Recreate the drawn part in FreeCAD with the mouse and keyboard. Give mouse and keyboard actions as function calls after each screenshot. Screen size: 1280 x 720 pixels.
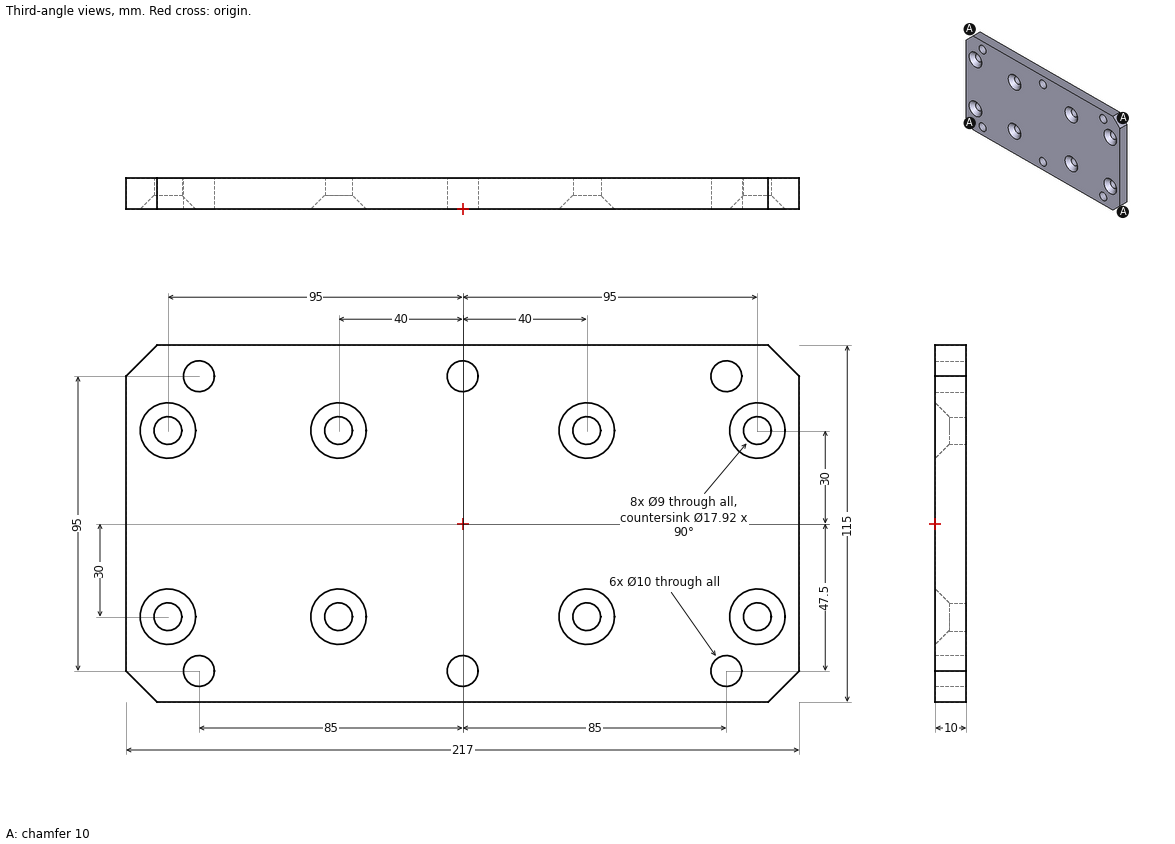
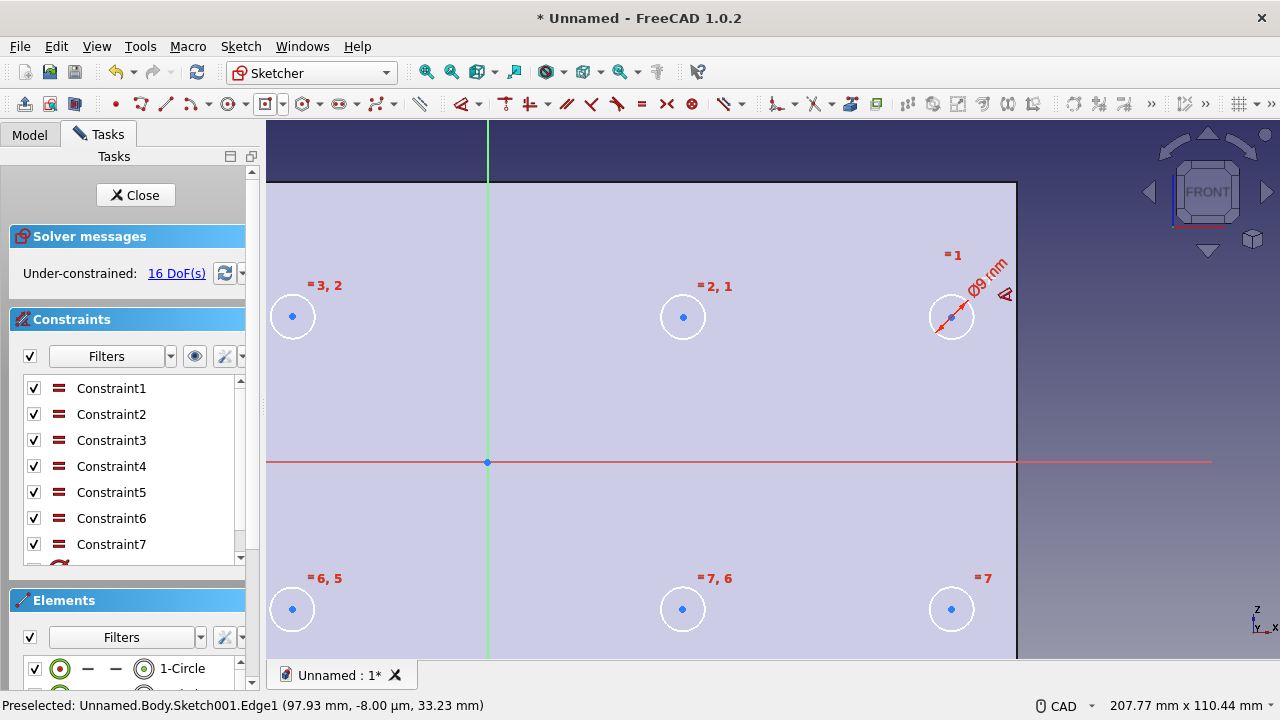
click(952, 317)
click(720, 283)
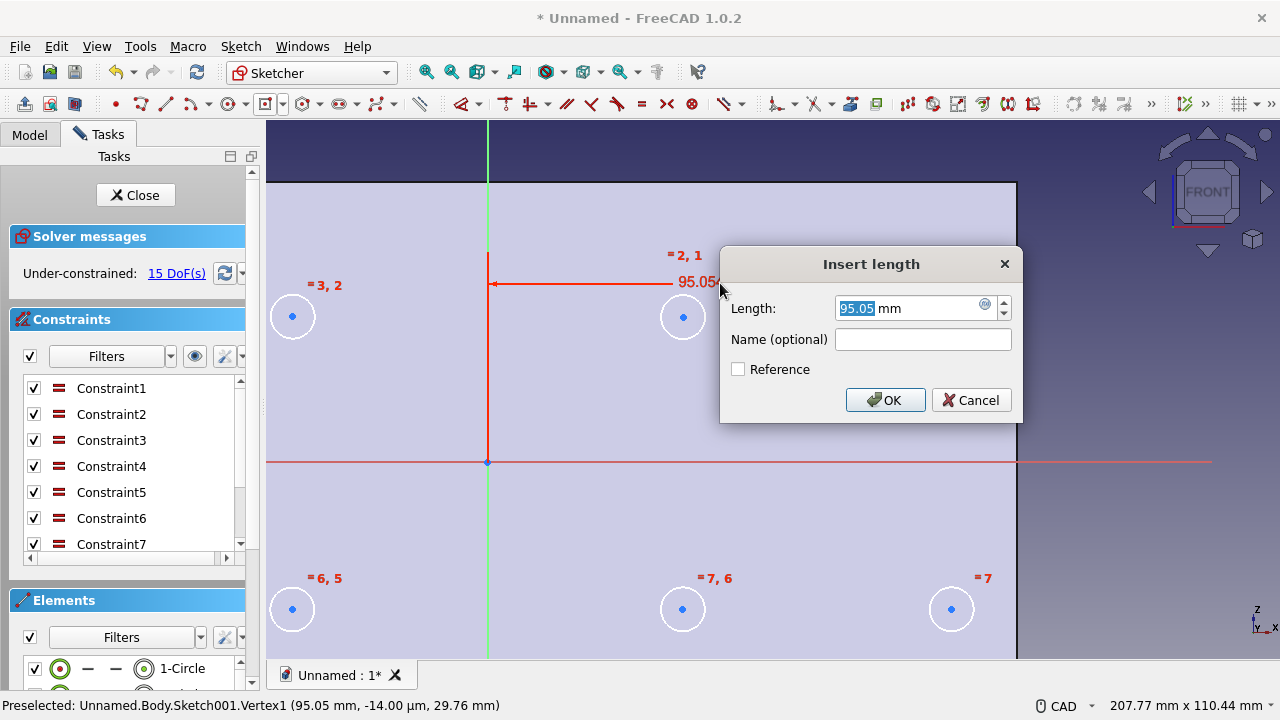
text(95)
key(Return)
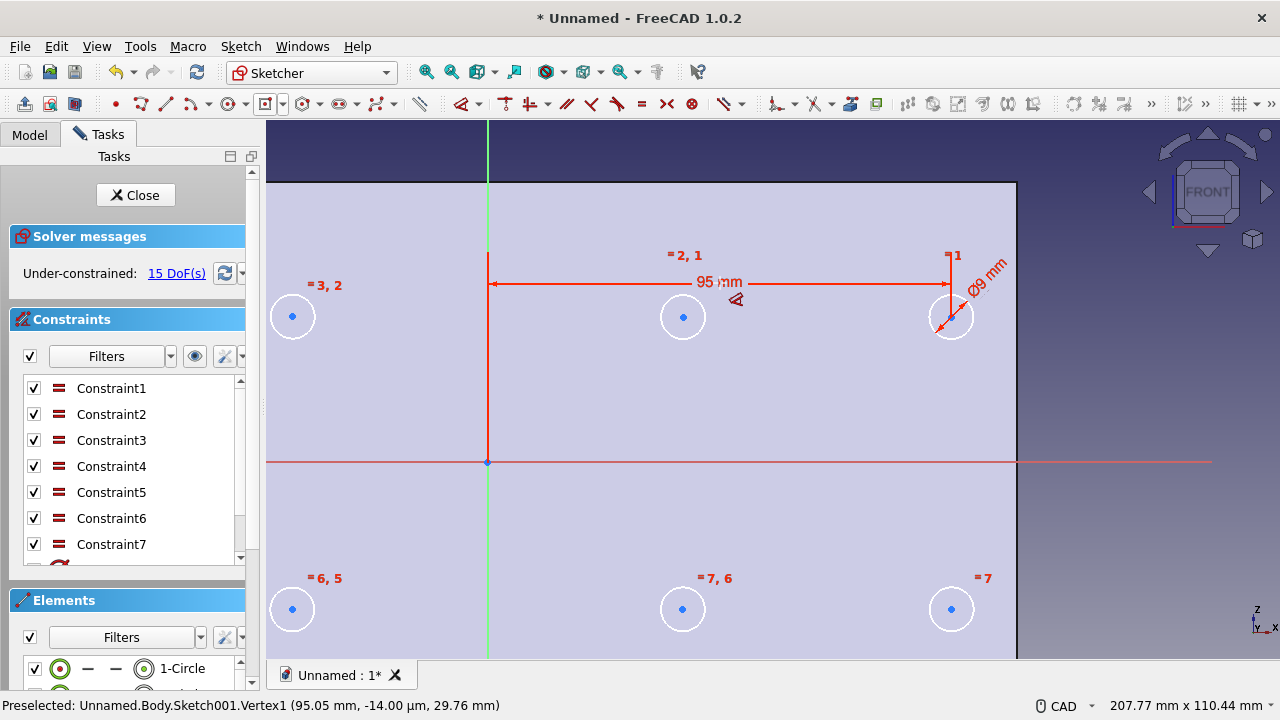
click(951, 317)
click(985, 390)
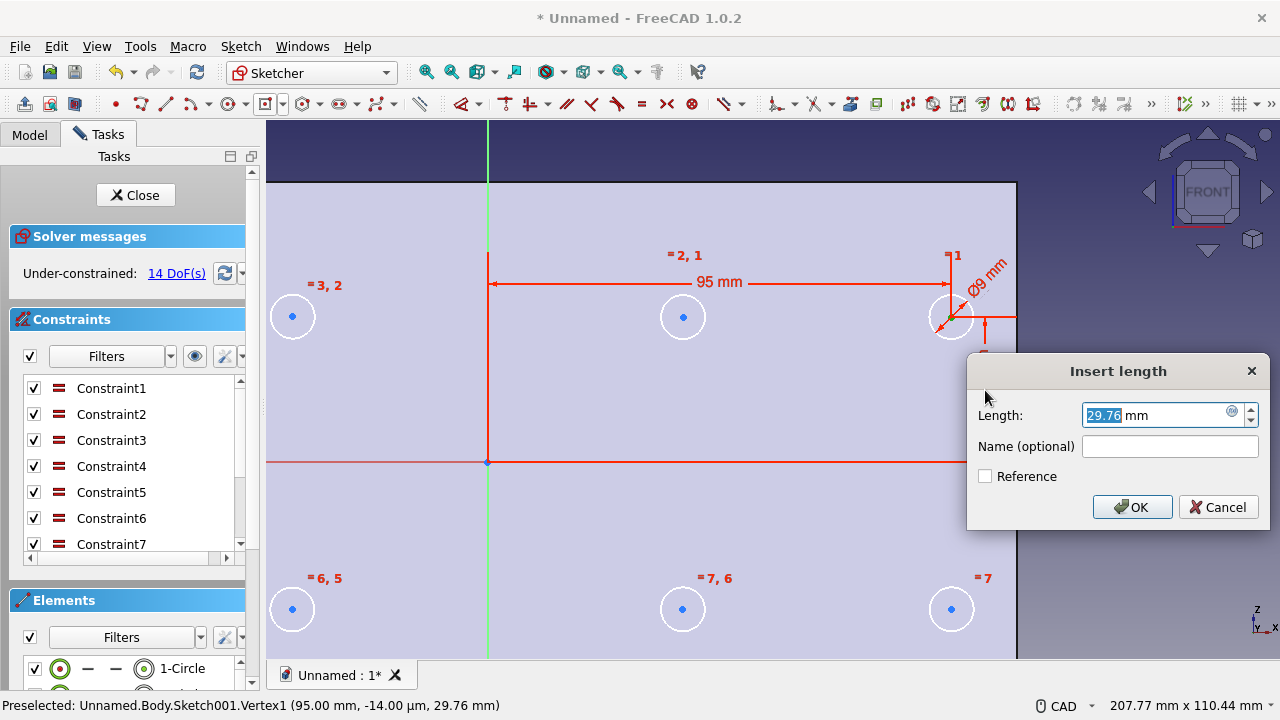
text(30)
key(Return)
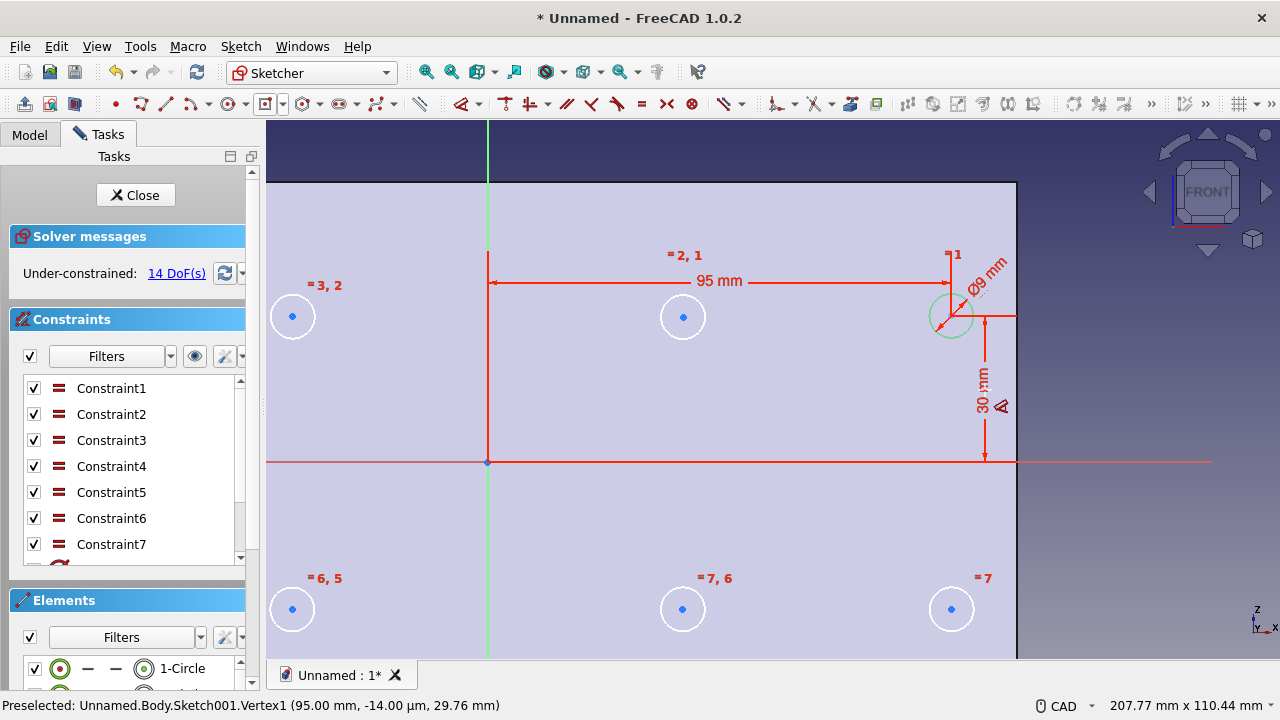
click(683, 317)
click(585, 283)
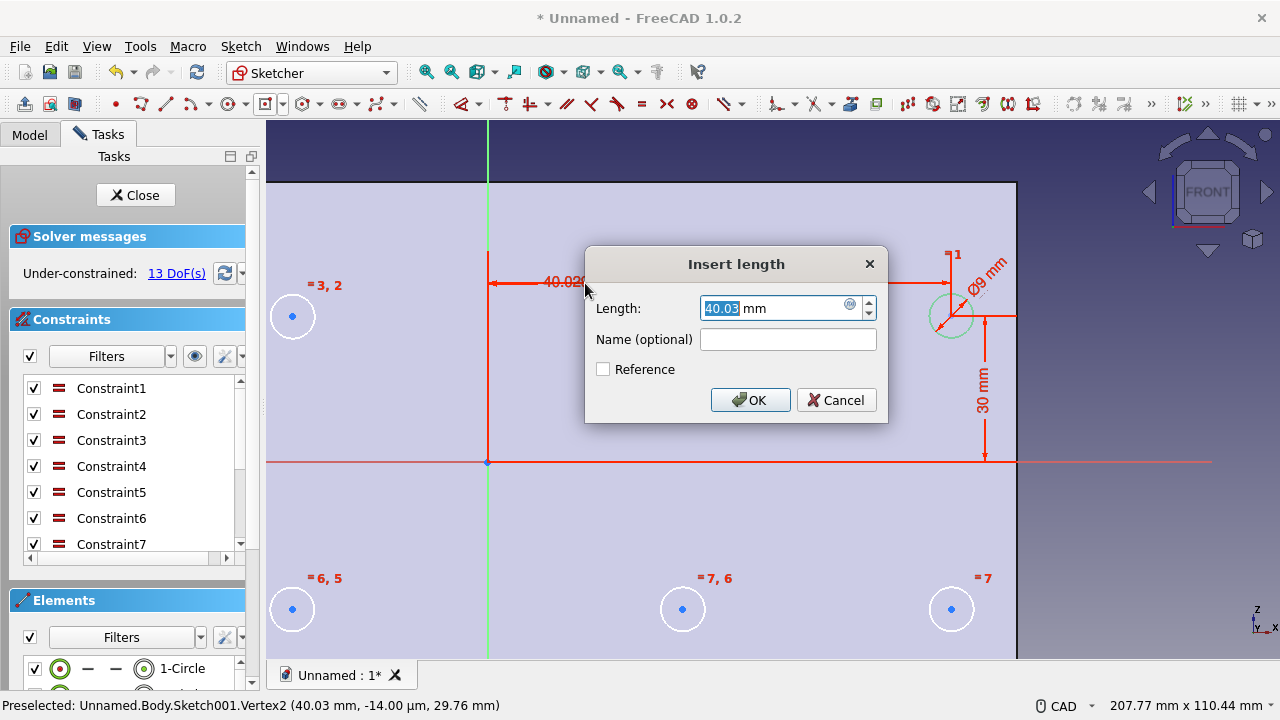
text(40)
key(Return)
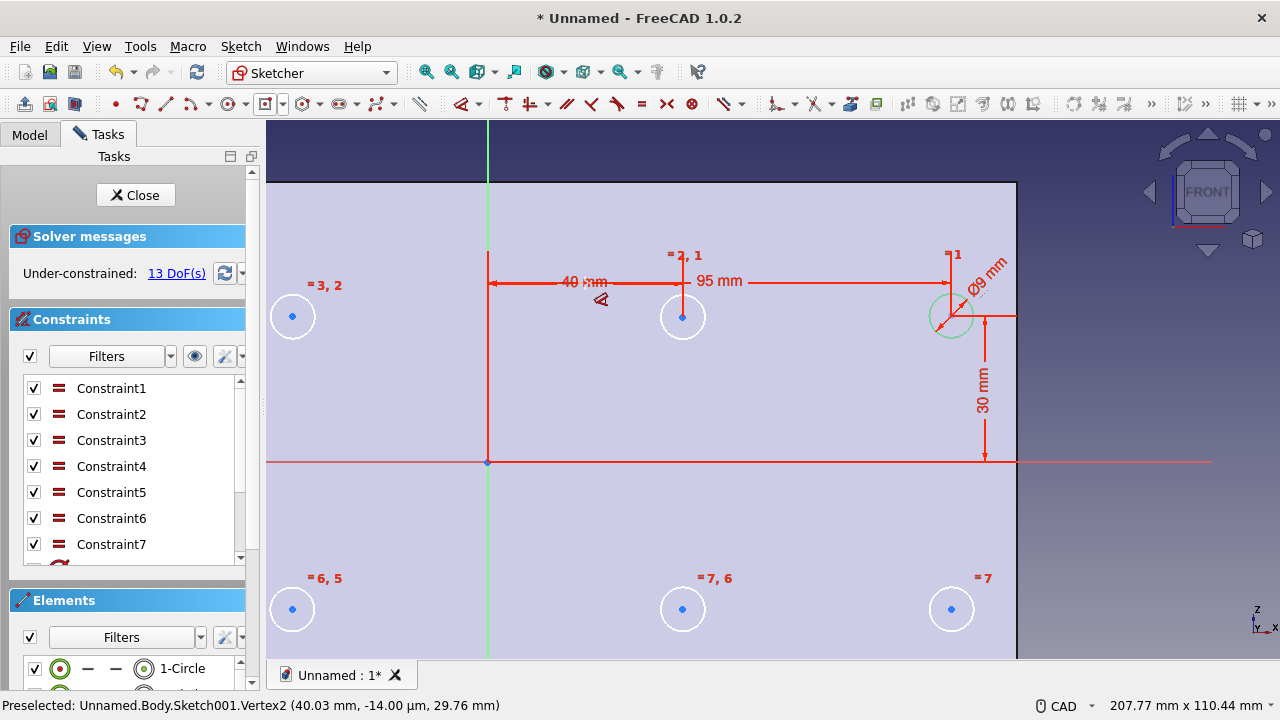
click(683, 317)
click(717, 390)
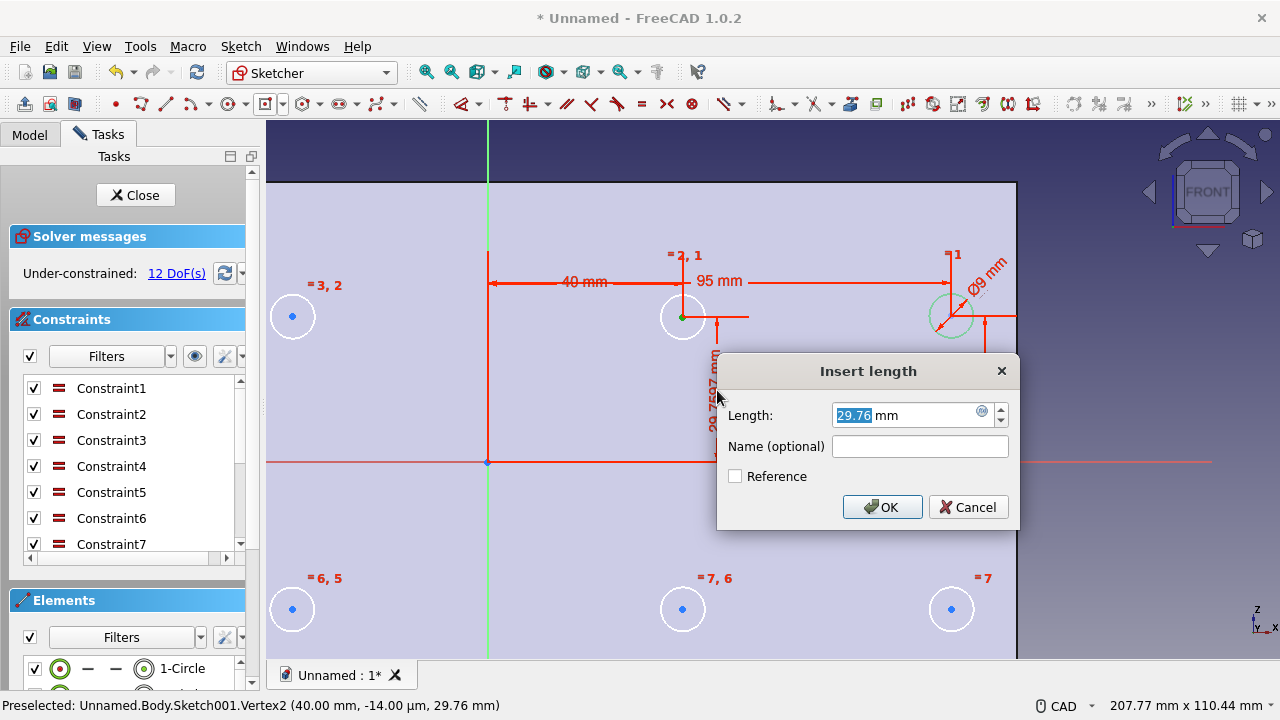
text(30)
key(Return)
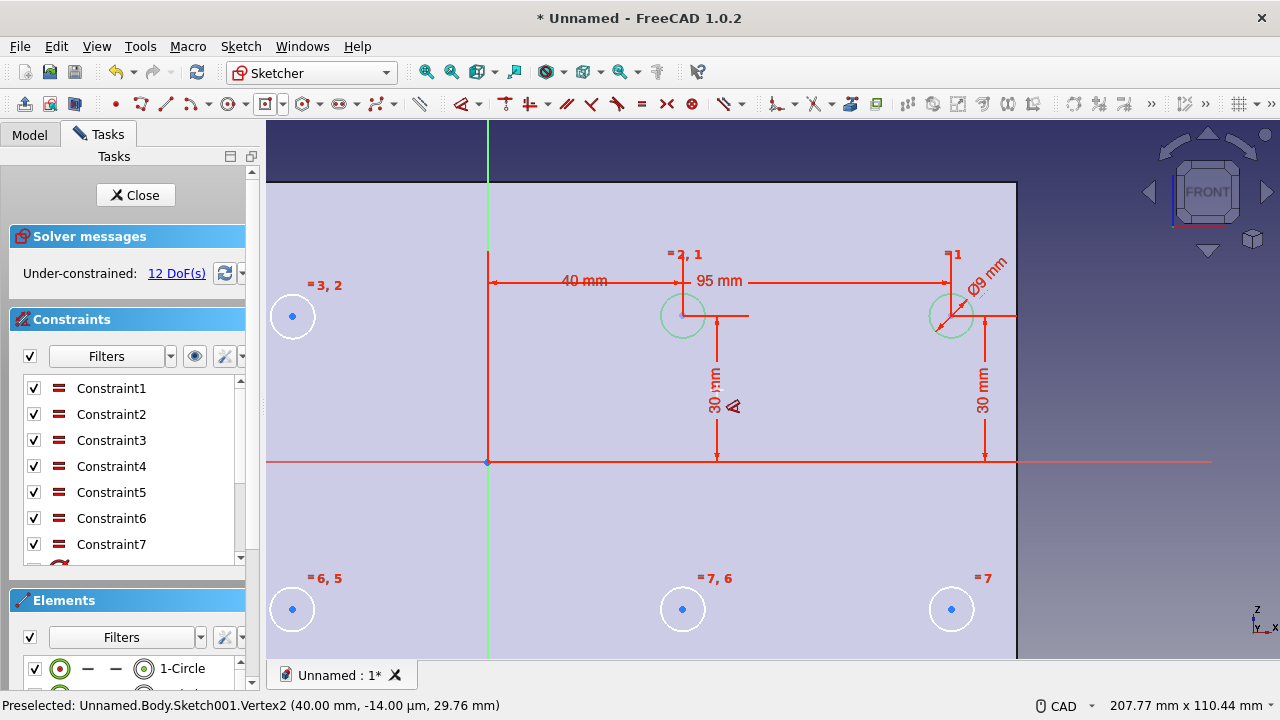
scroll(968, 301, down, 3)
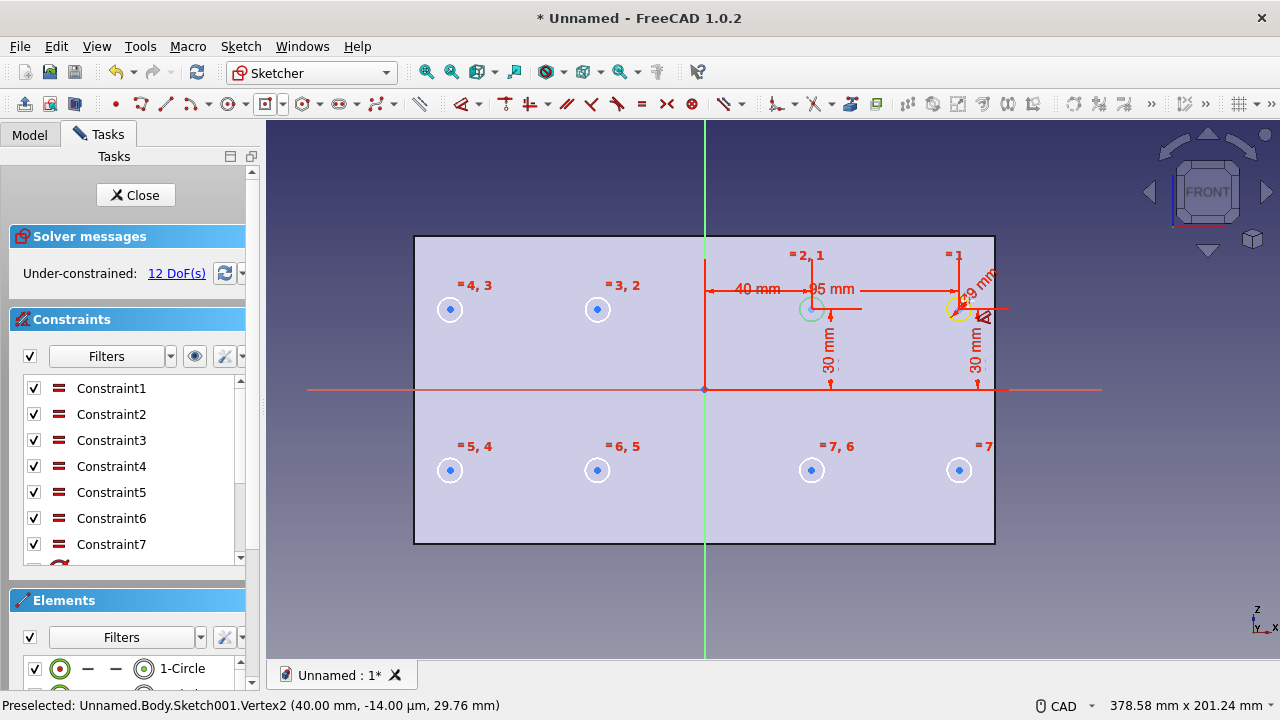
click(598, 310)
click(651, 276)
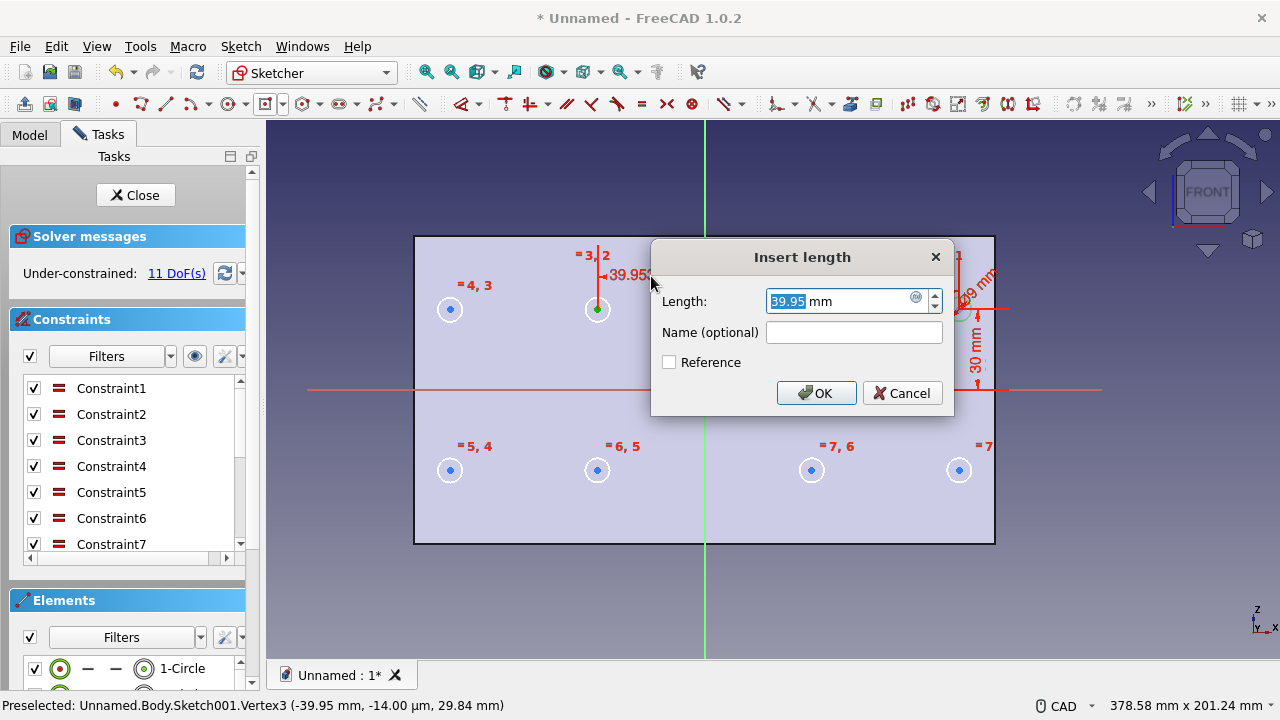
text(40)
key(Return)